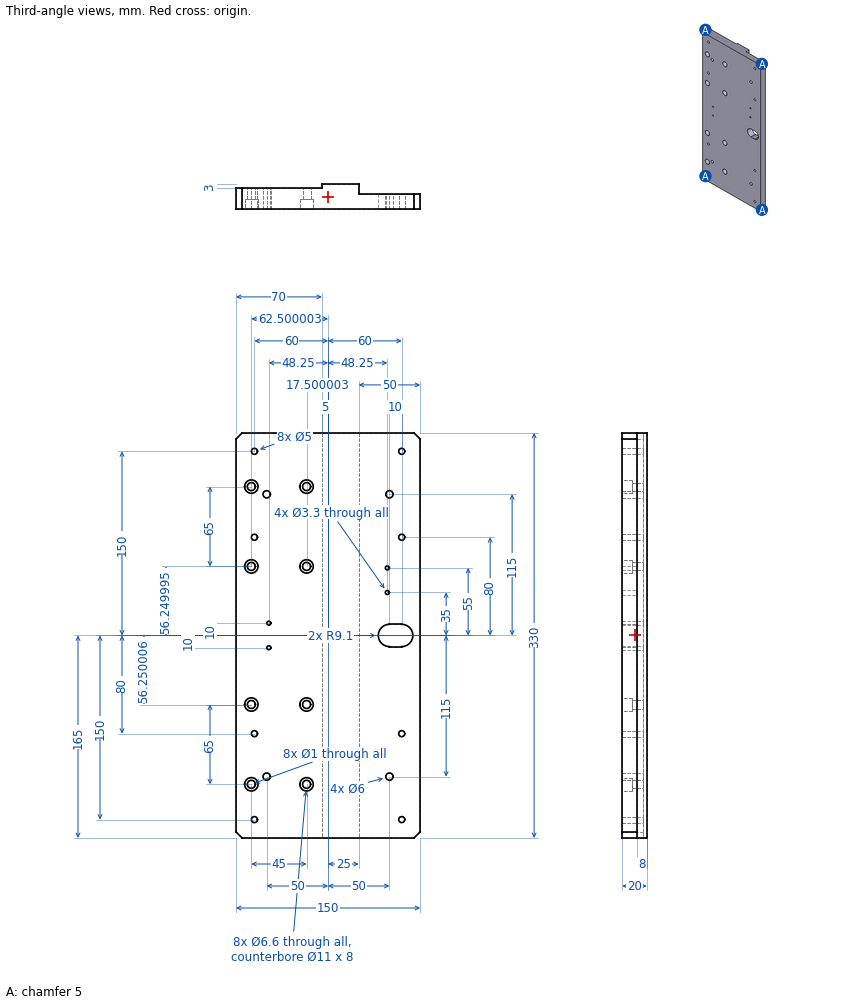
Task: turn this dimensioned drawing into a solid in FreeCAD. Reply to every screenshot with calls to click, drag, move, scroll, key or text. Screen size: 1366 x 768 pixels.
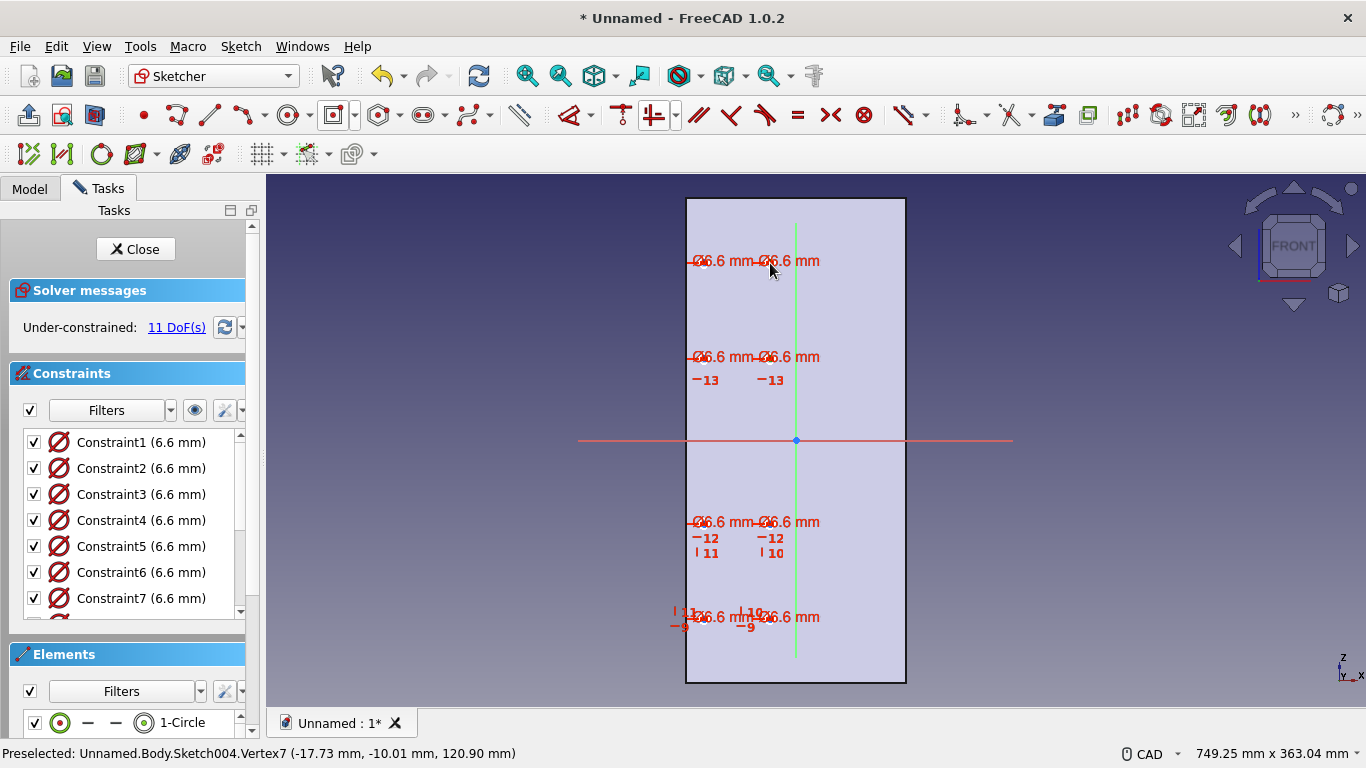
click(676, 116)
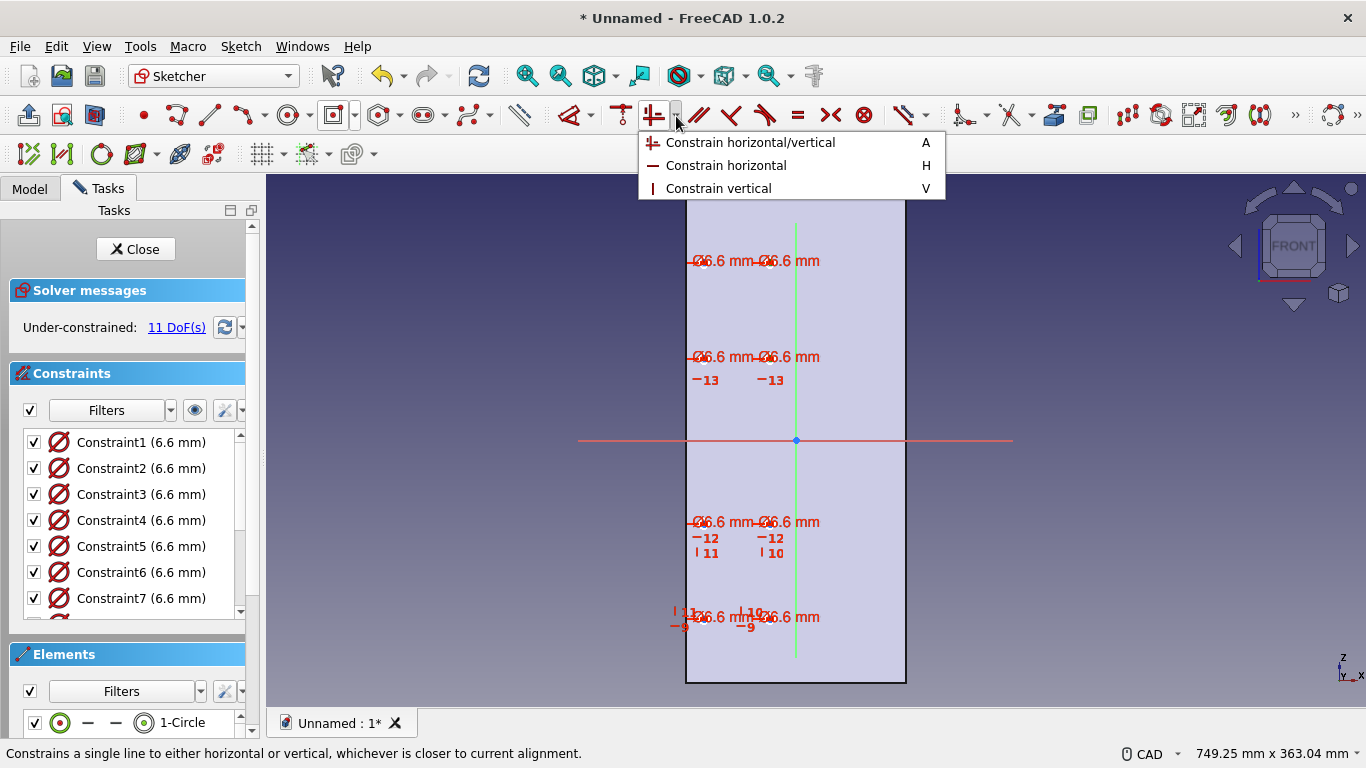
click(792, 188)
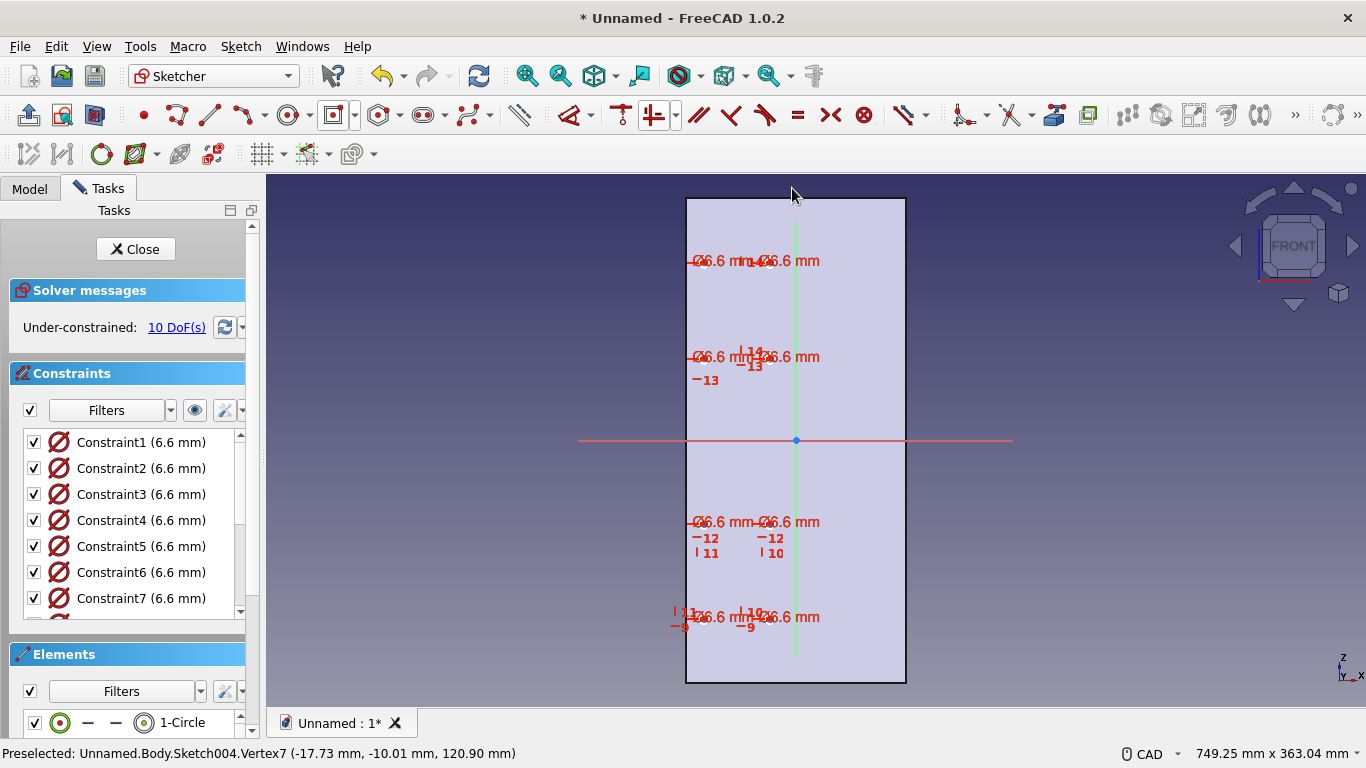
click(704, 359)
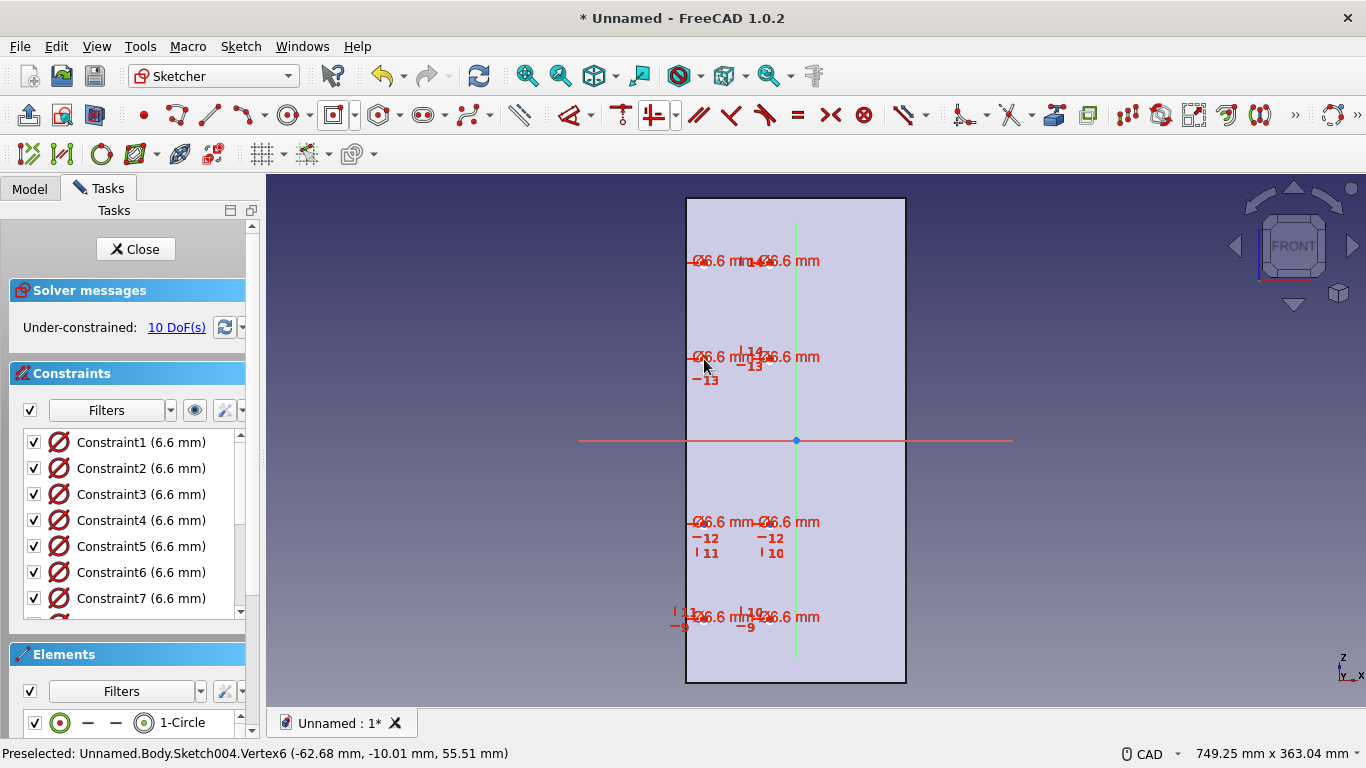
click(704, 263)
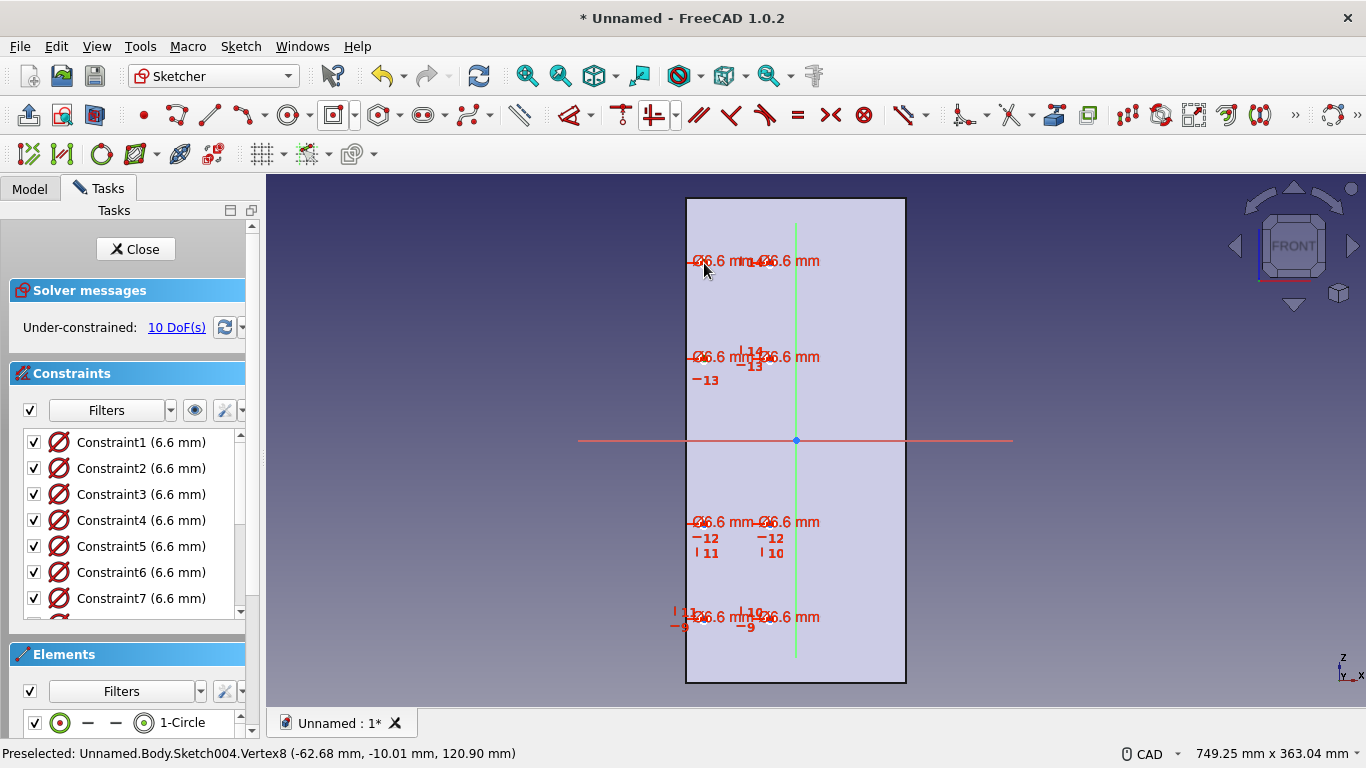
click(676, 116)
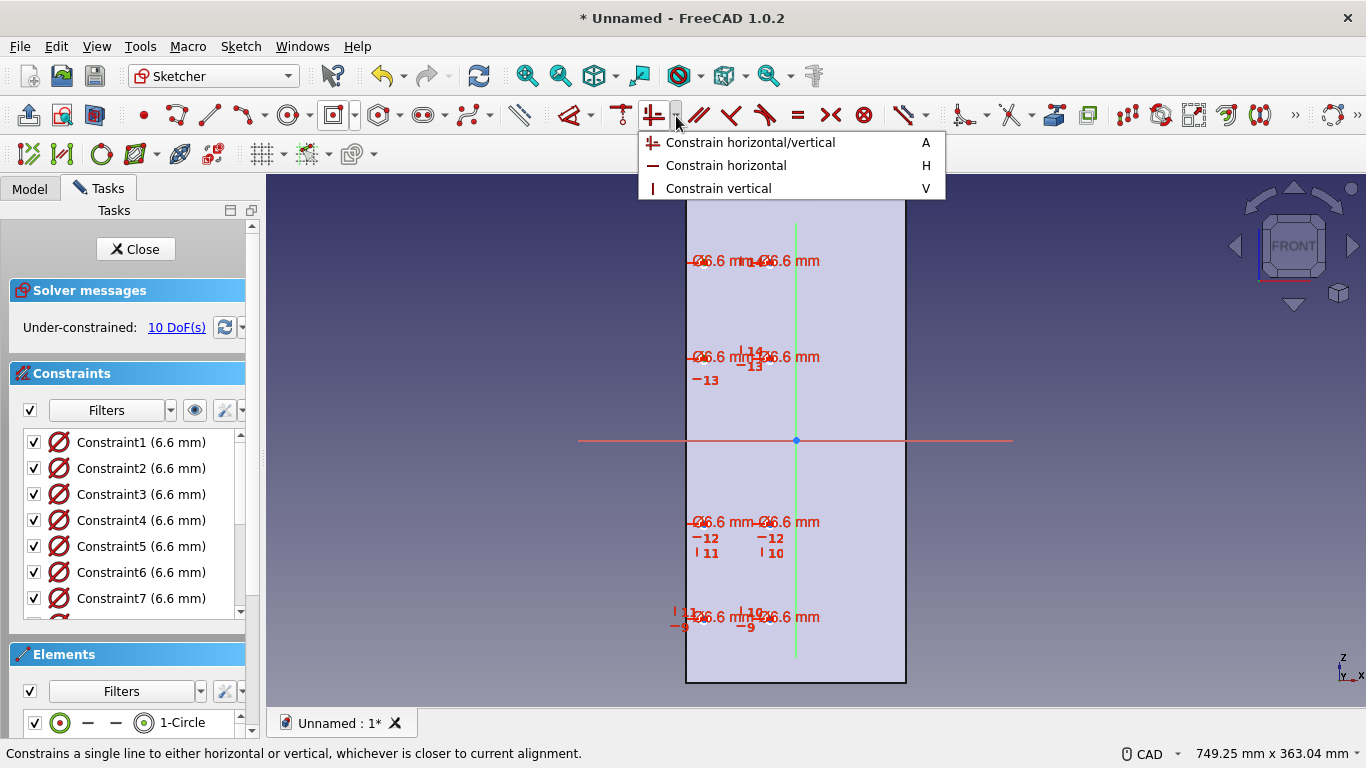
click(792, 188)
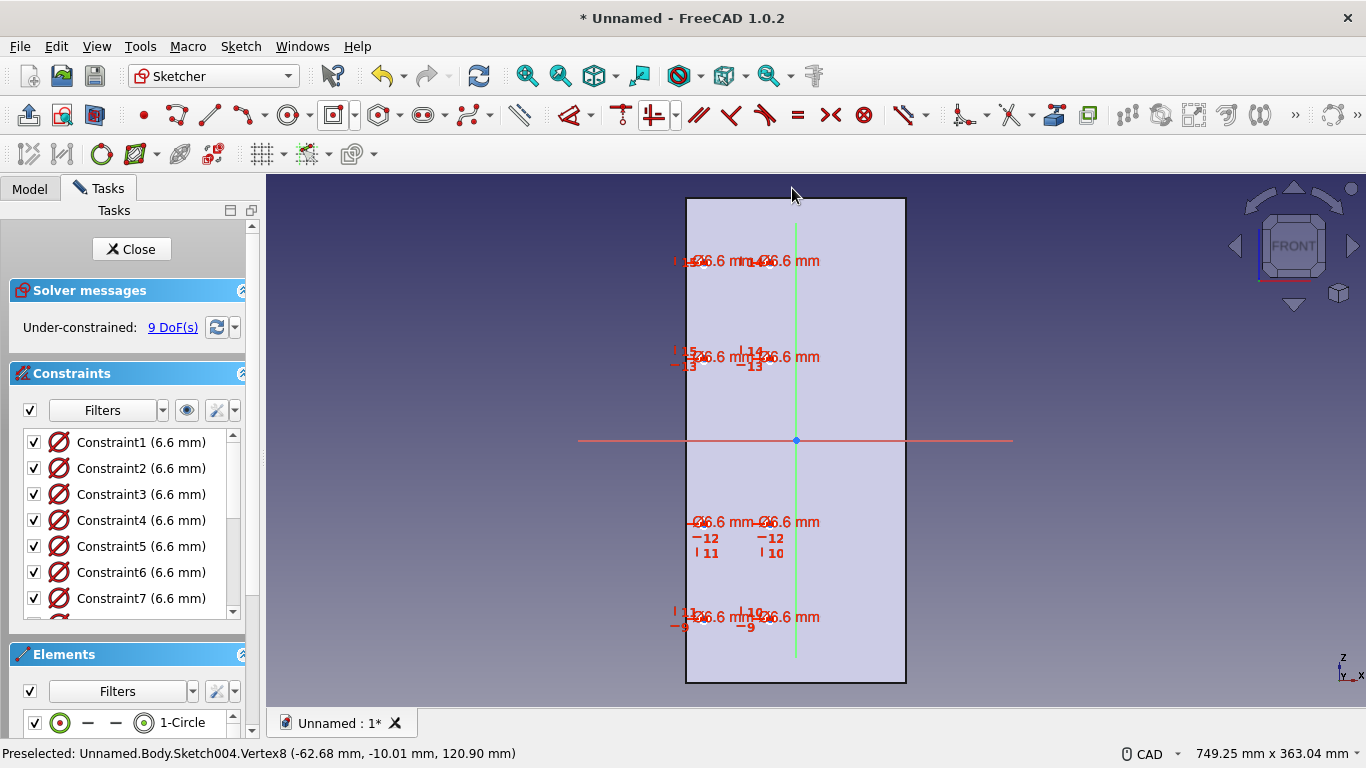
click(770, 263)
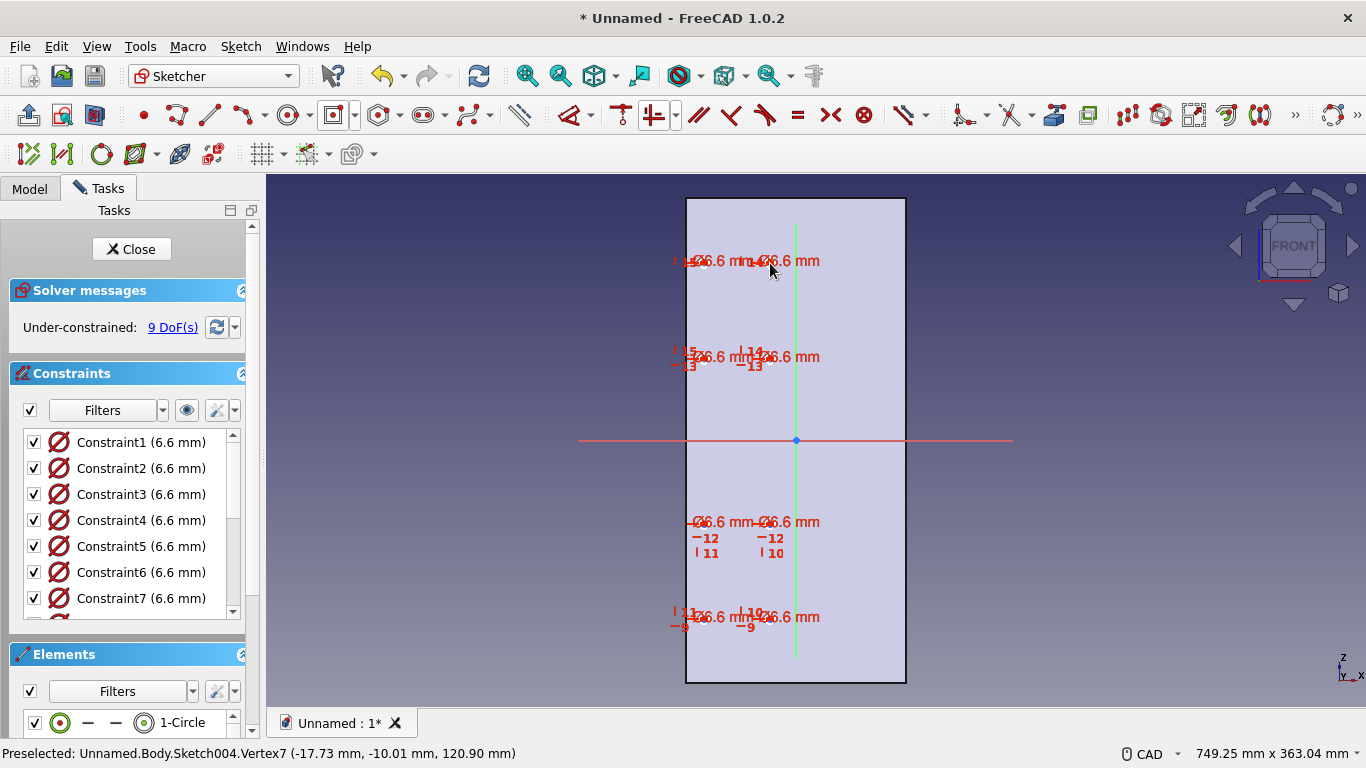
click(704, 263)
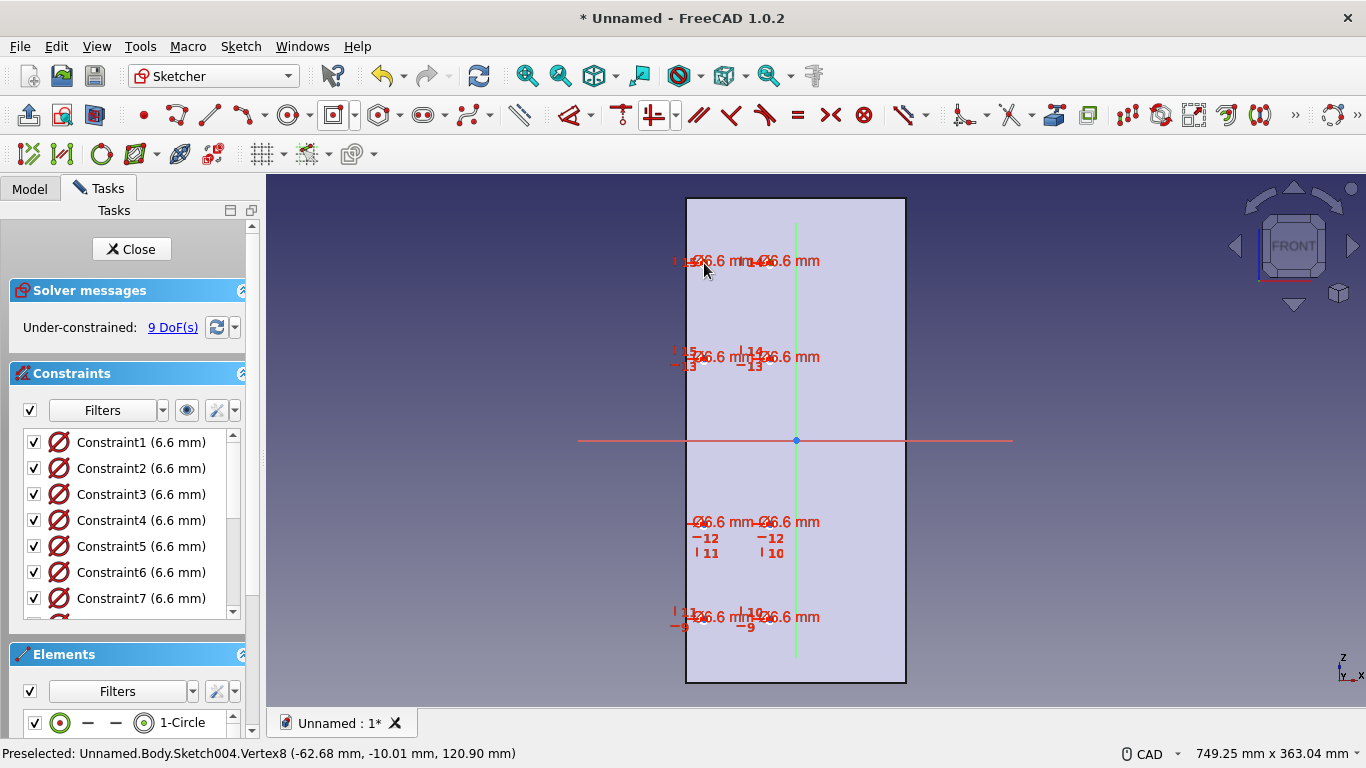
key(h)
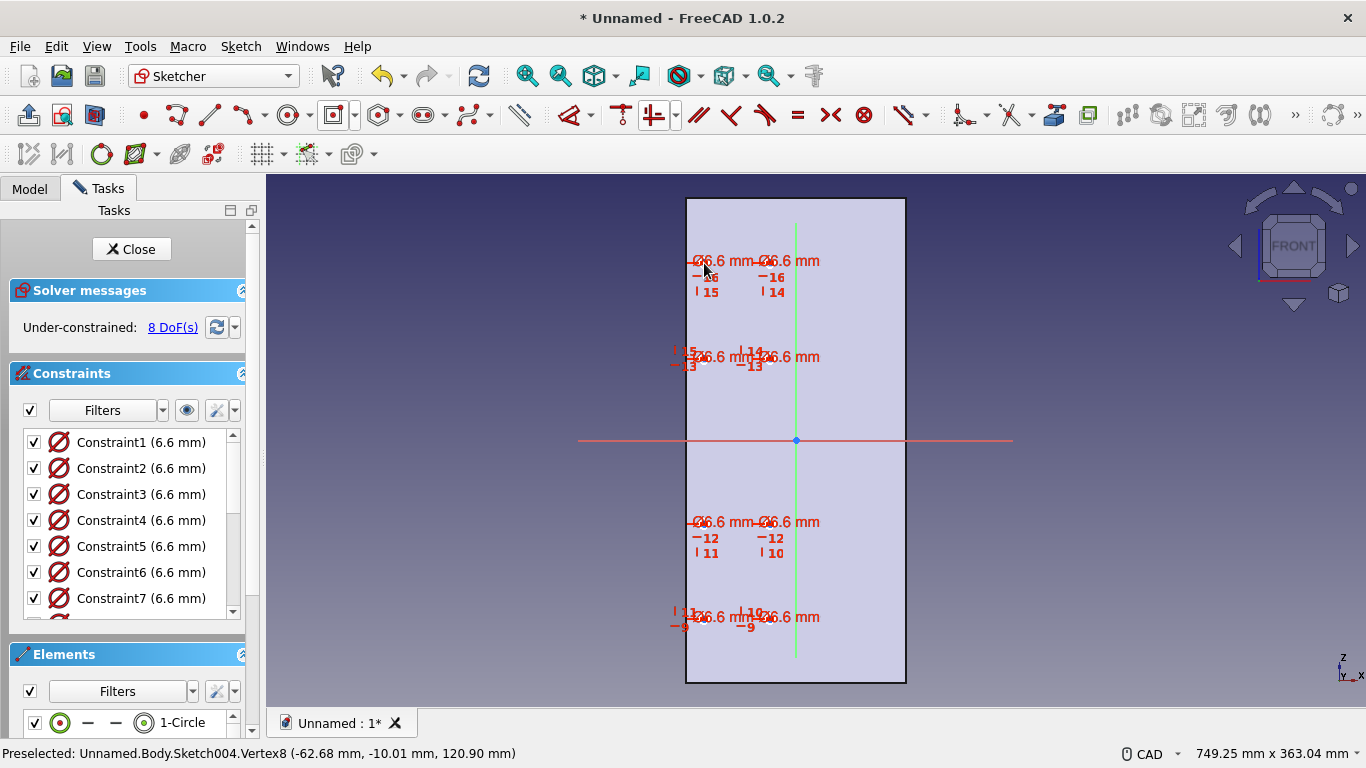
click(568, 116)